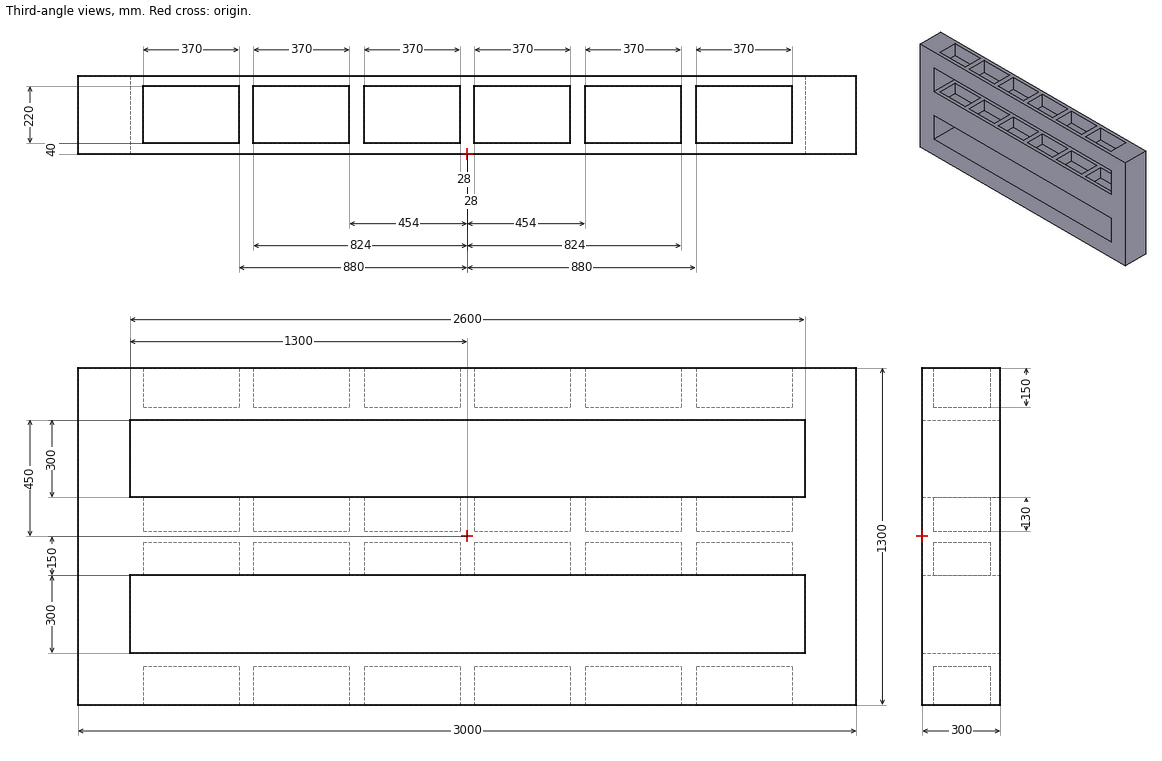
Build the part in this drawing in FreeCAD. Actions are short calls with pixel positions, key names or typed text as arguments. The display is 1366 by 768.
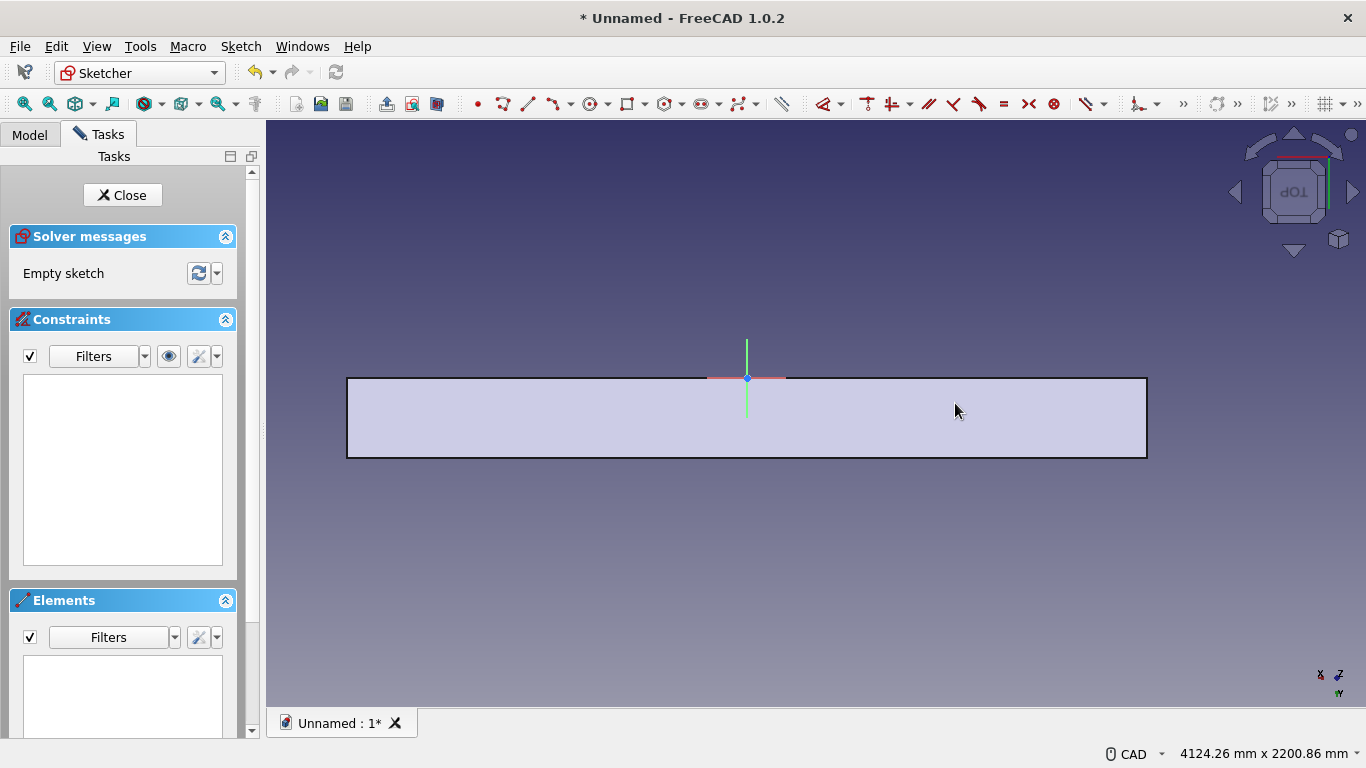
key(g)
key(r)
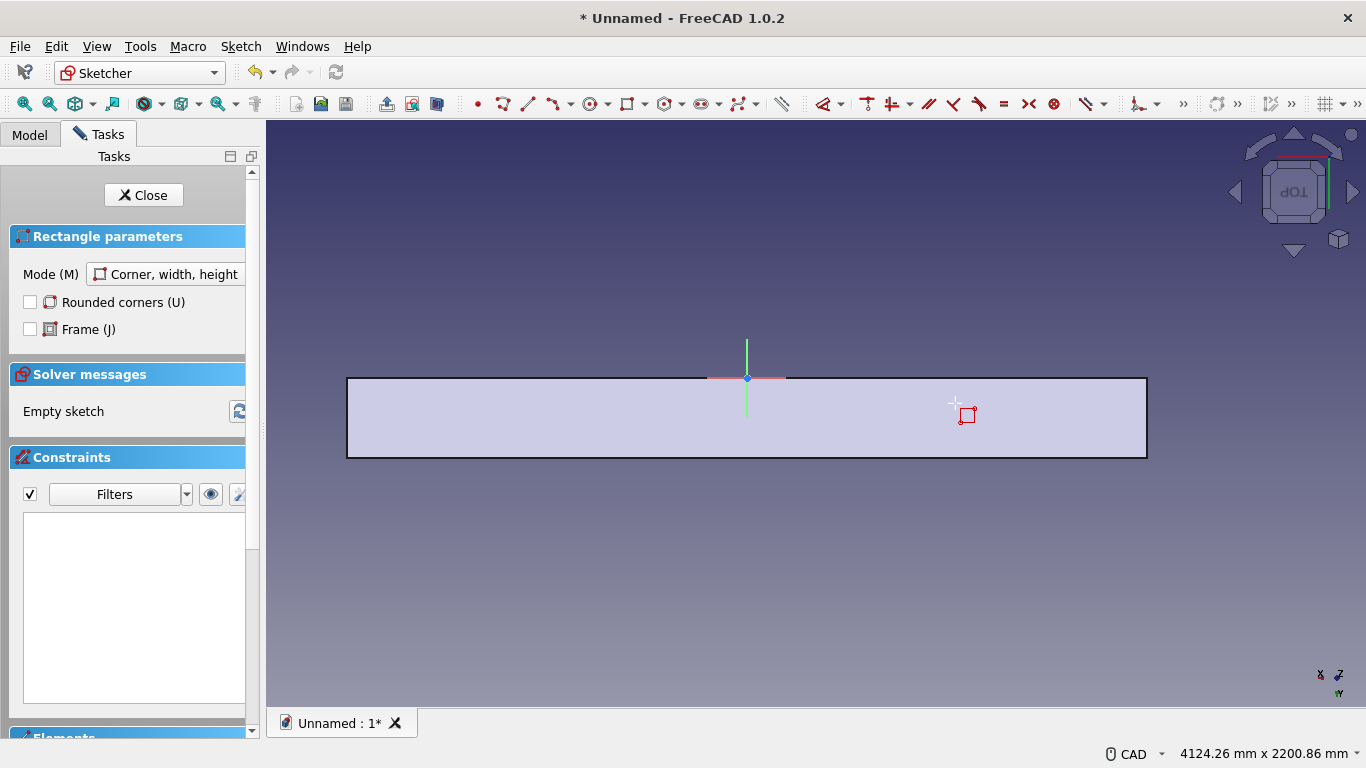
scroll(982, 389, up, 2)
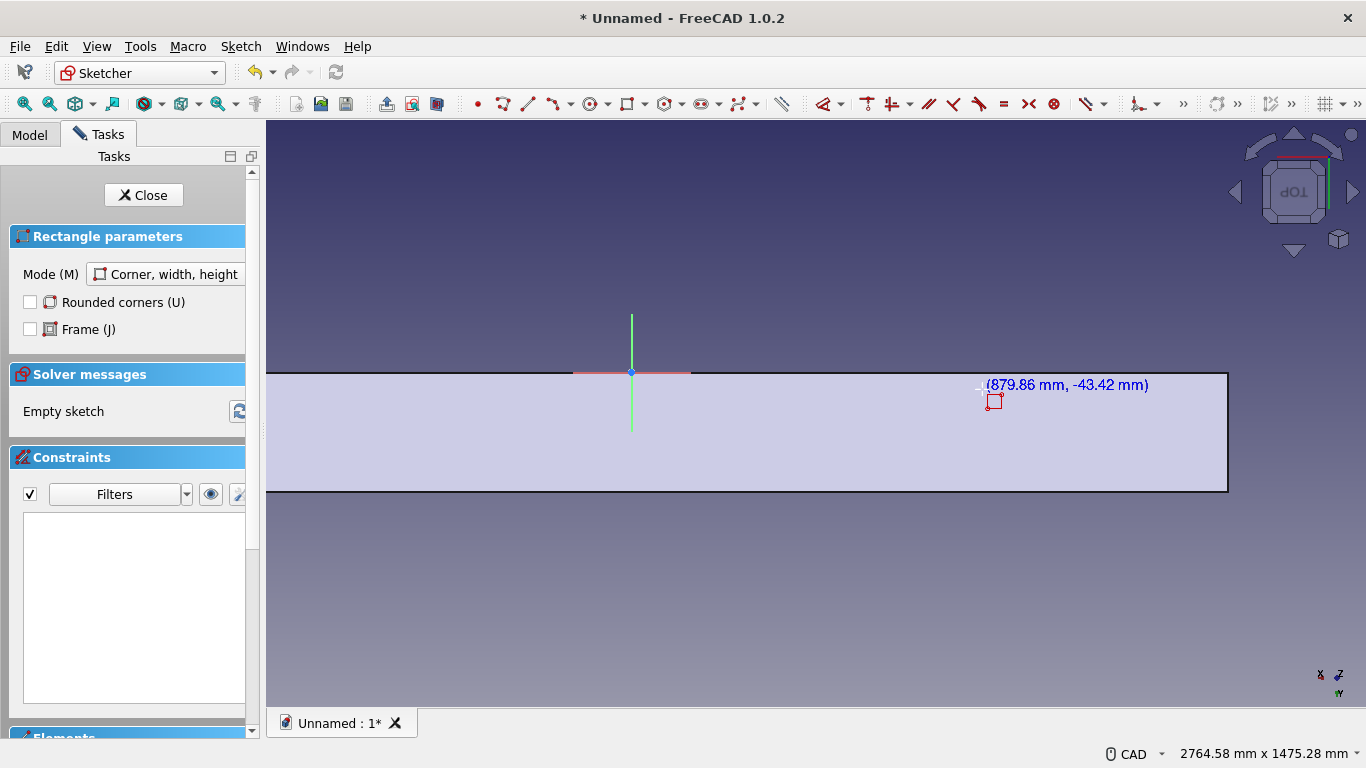
click(982, 389)
click(1129, 476)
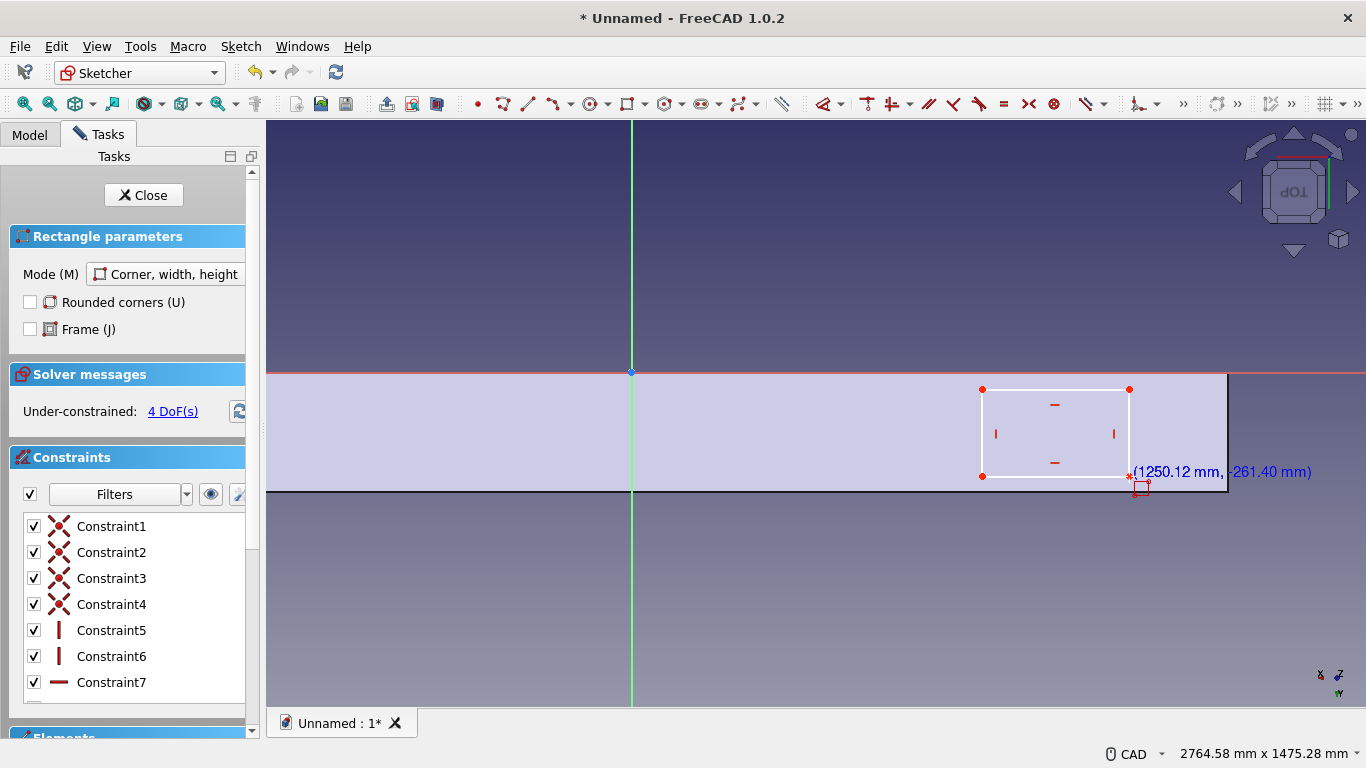
scroll(983, 391, down, 2)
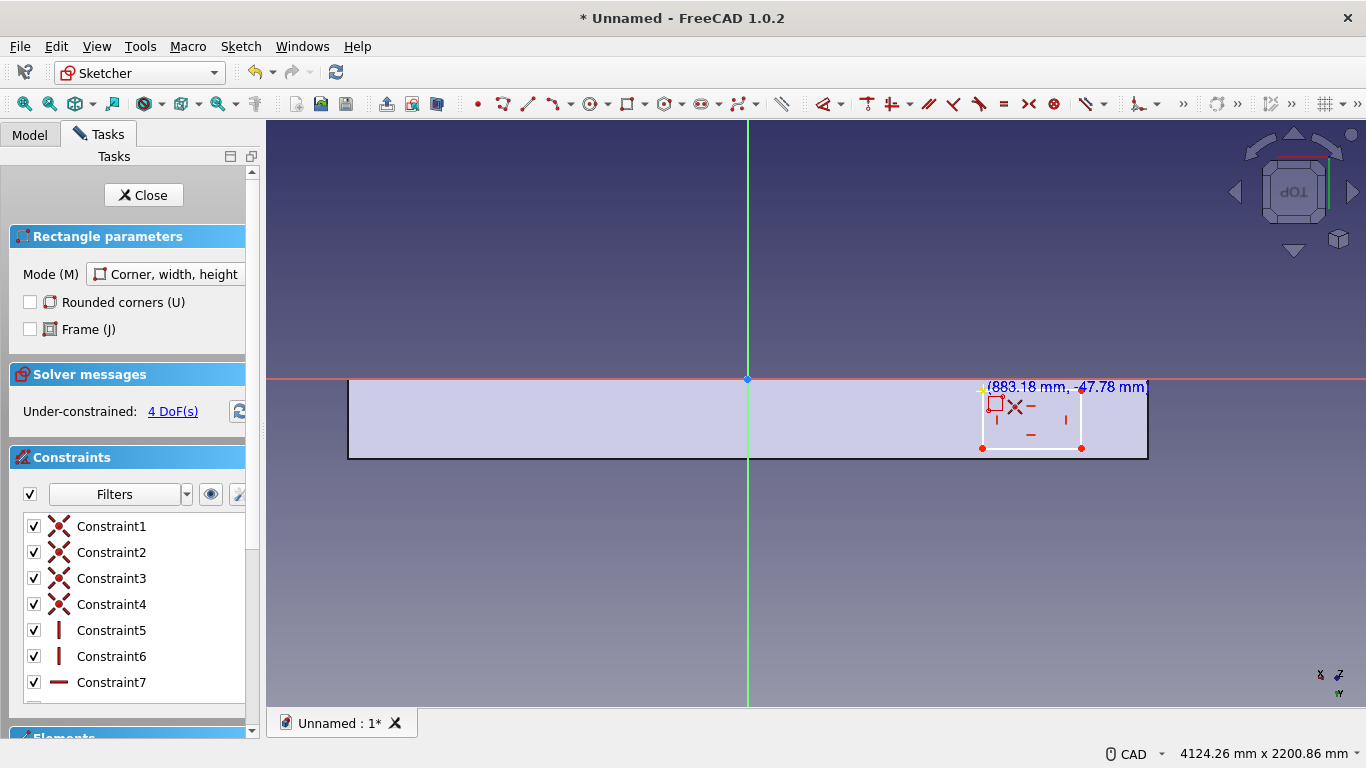
scroll(414, 390, up, 2)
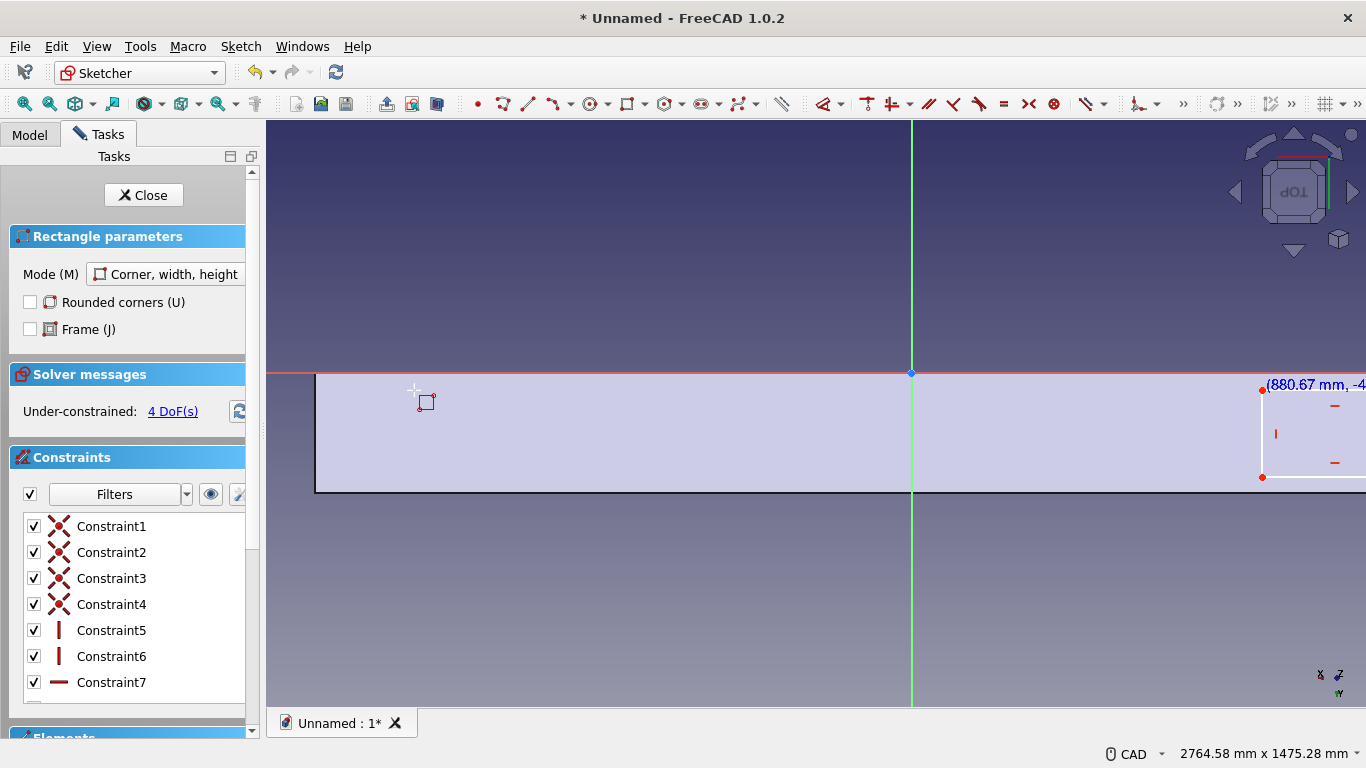
click(414, 389)
click(562, 477)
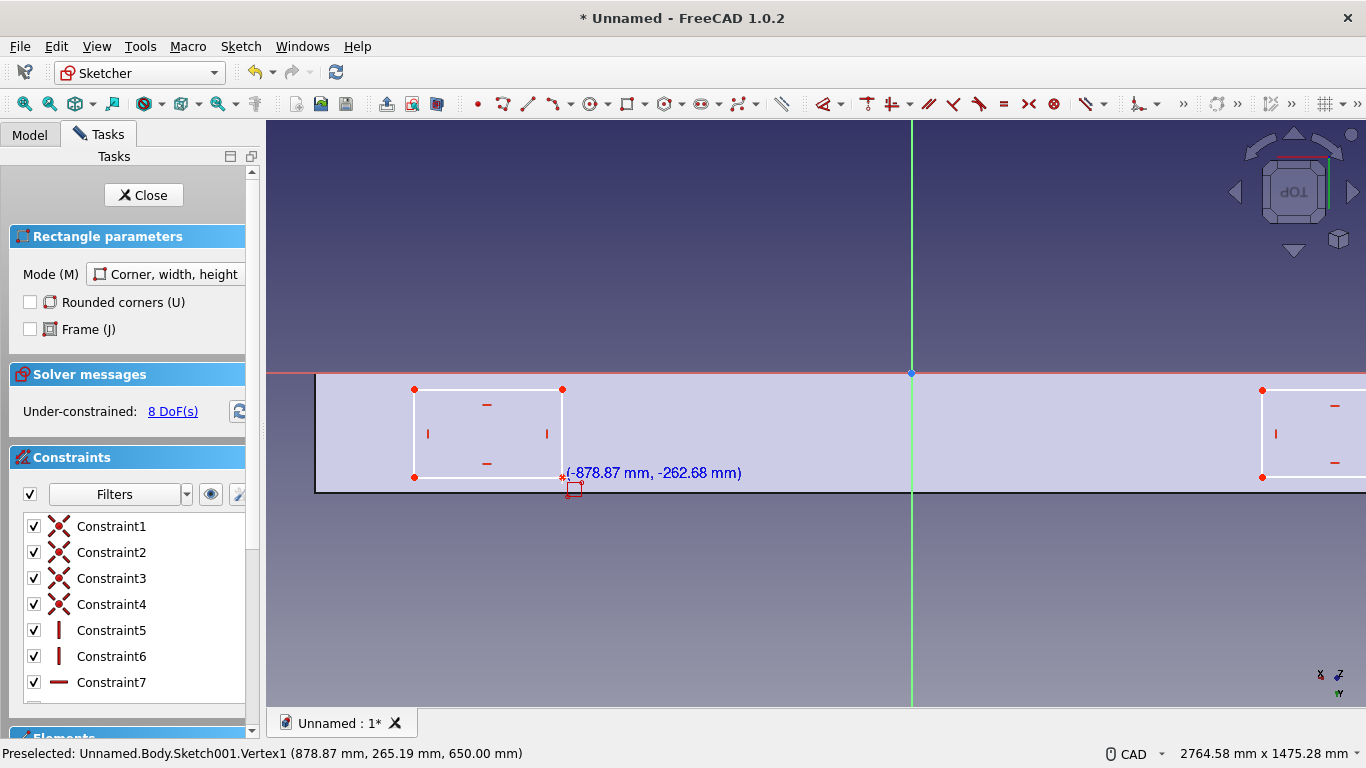
click(1092, 389)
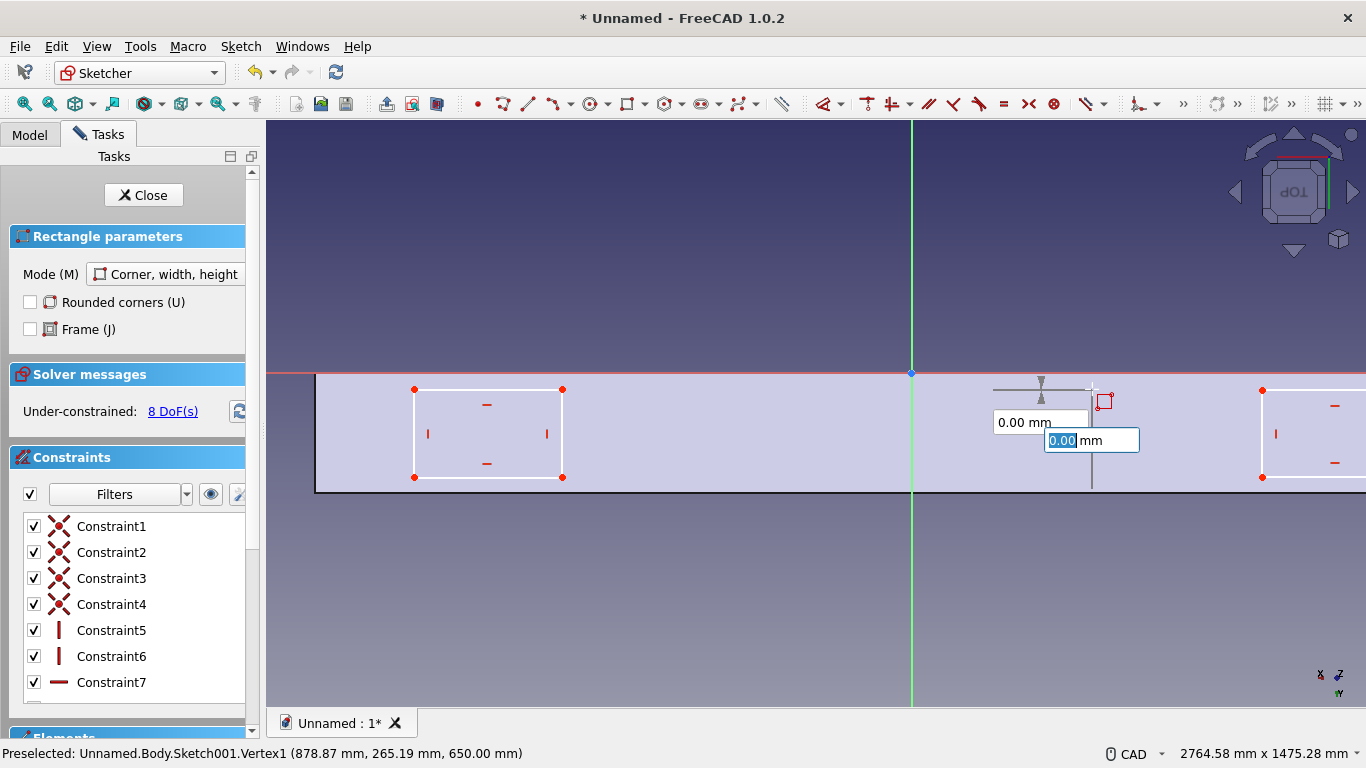
scroll(414, 390, down, 2)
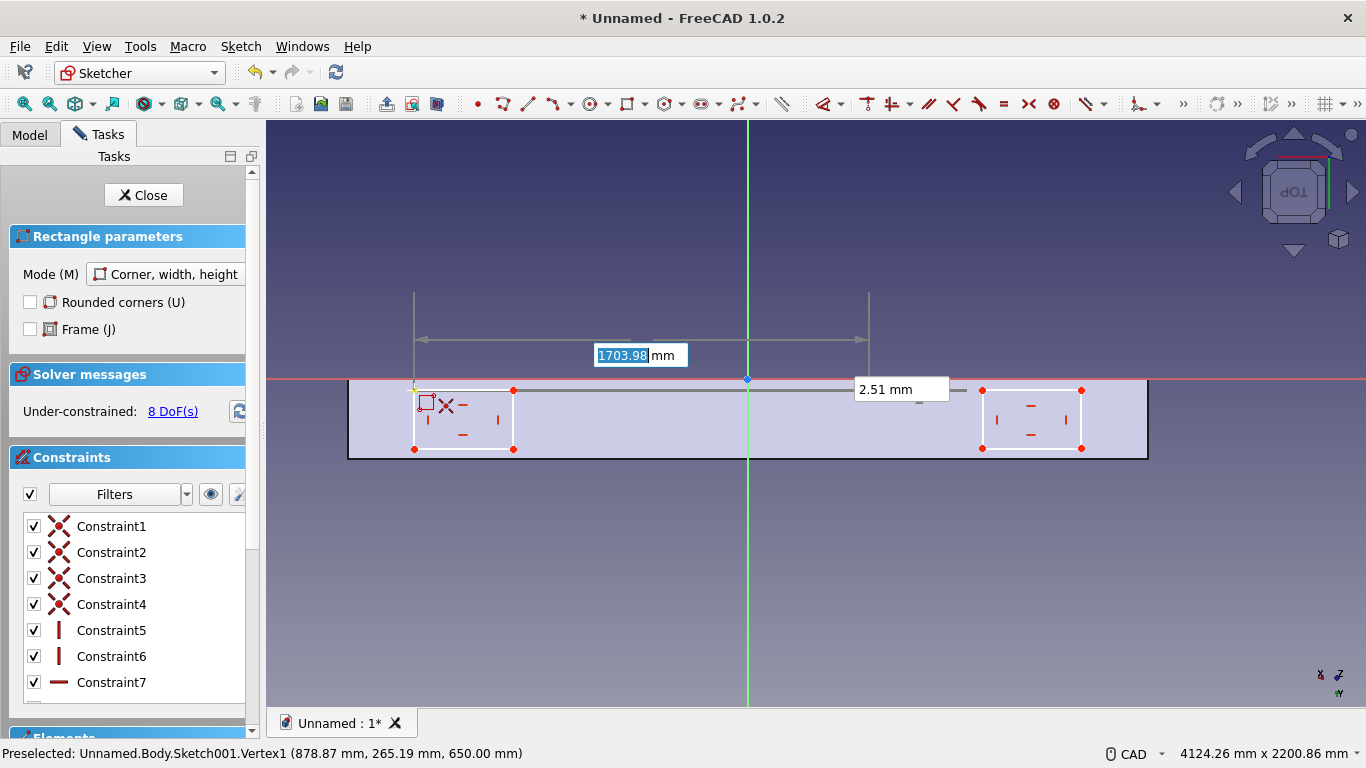
click(967, 448)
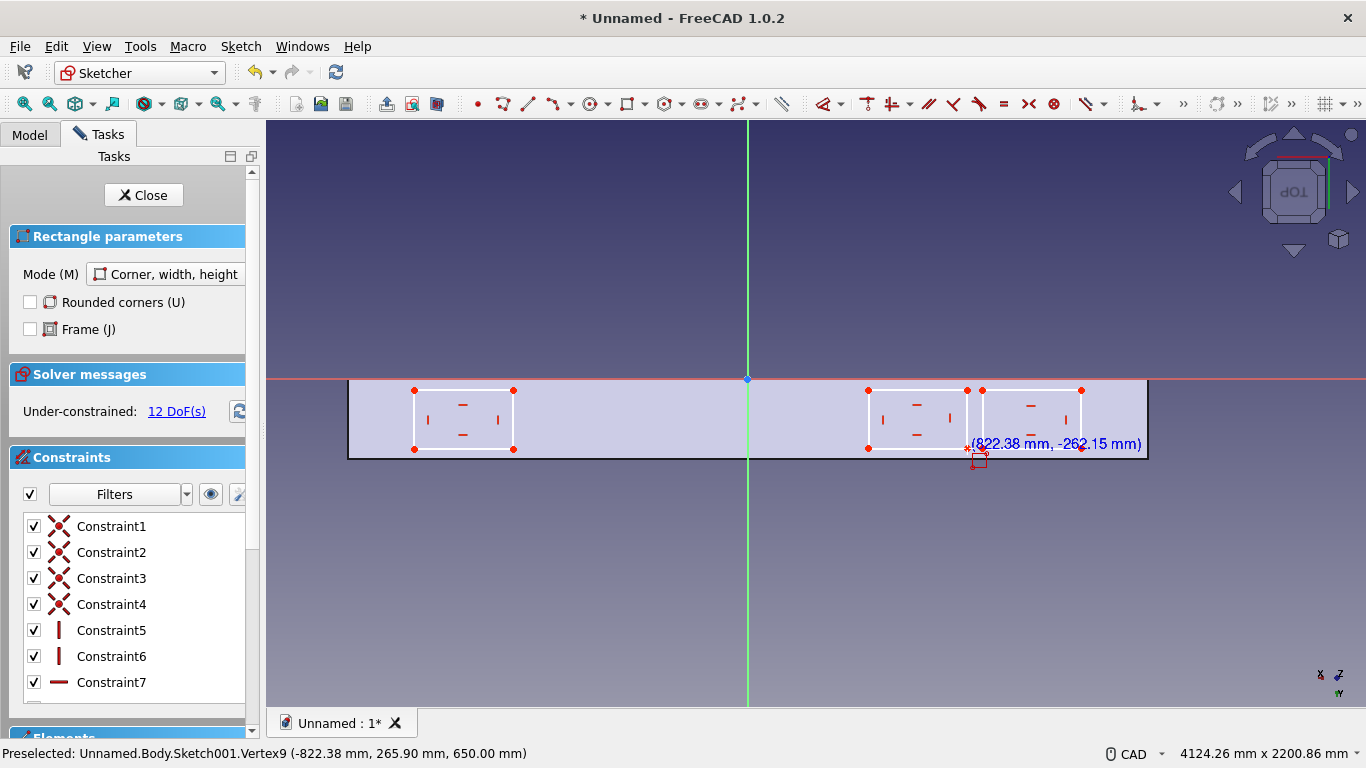
scroll(755, 390, up, 4)